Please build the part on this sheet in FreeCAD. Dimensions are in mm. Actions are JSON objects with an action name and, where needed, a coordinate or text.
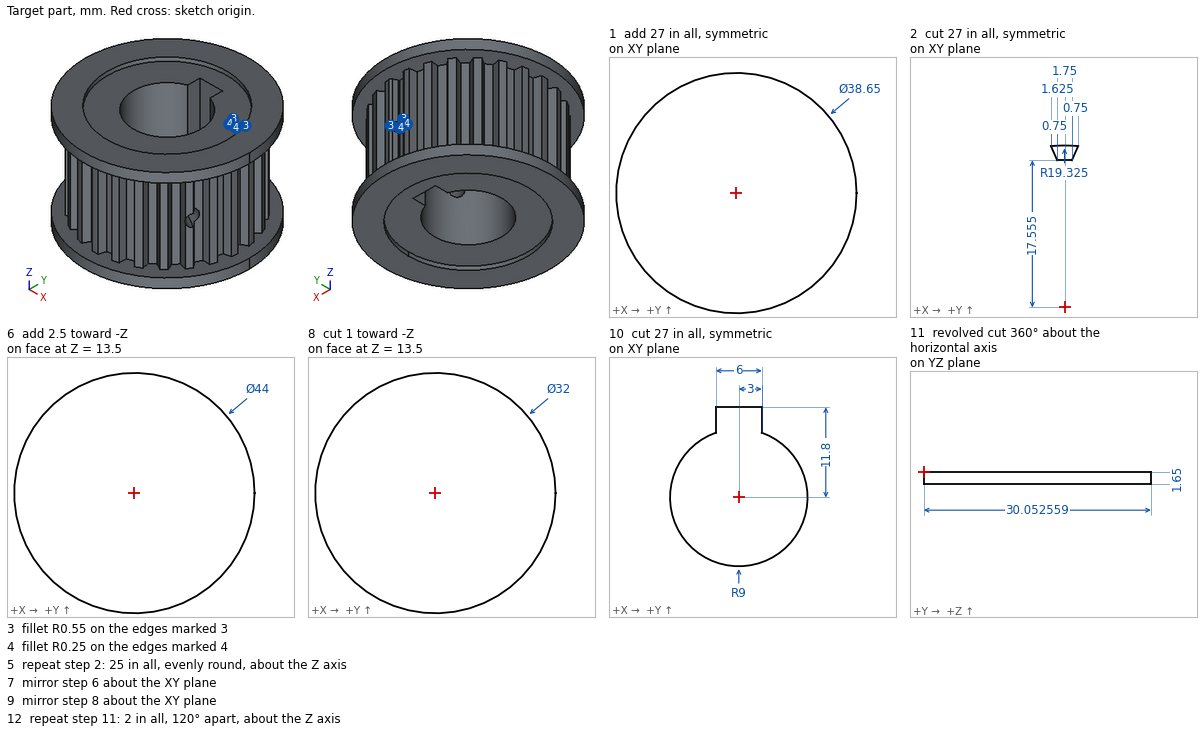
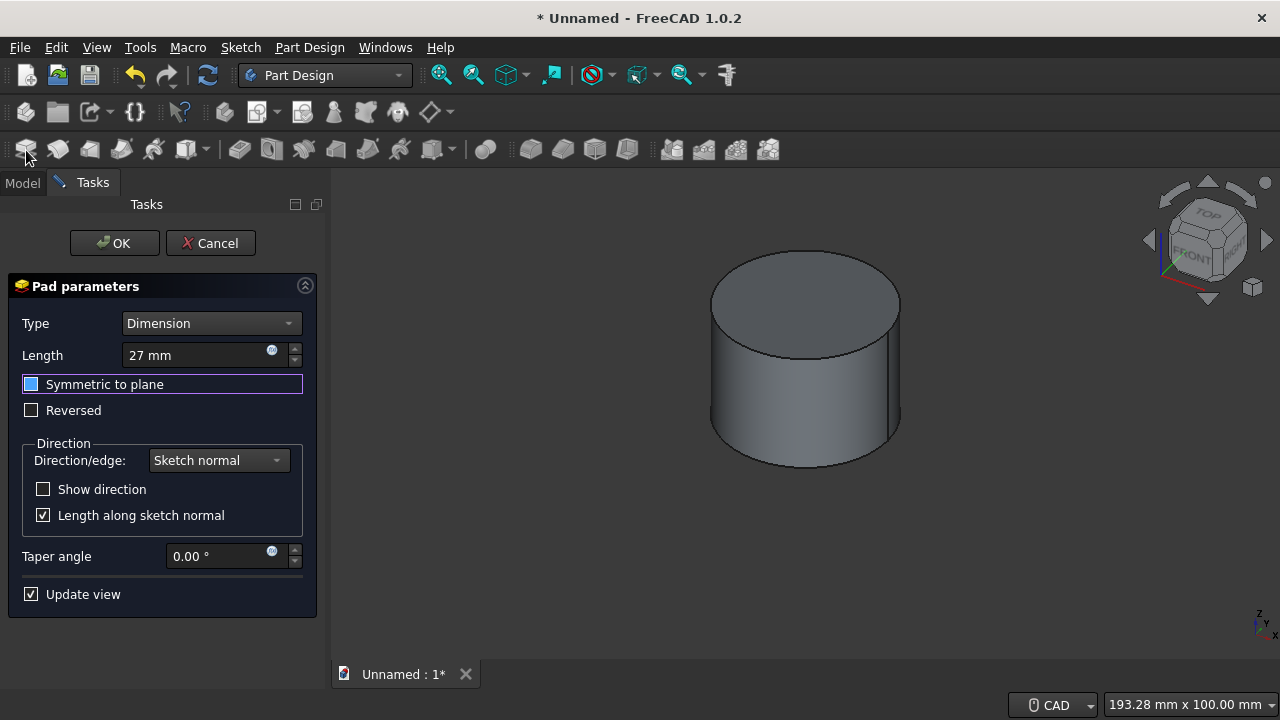
{"action": "left_click", "coordinate": [30, 384]}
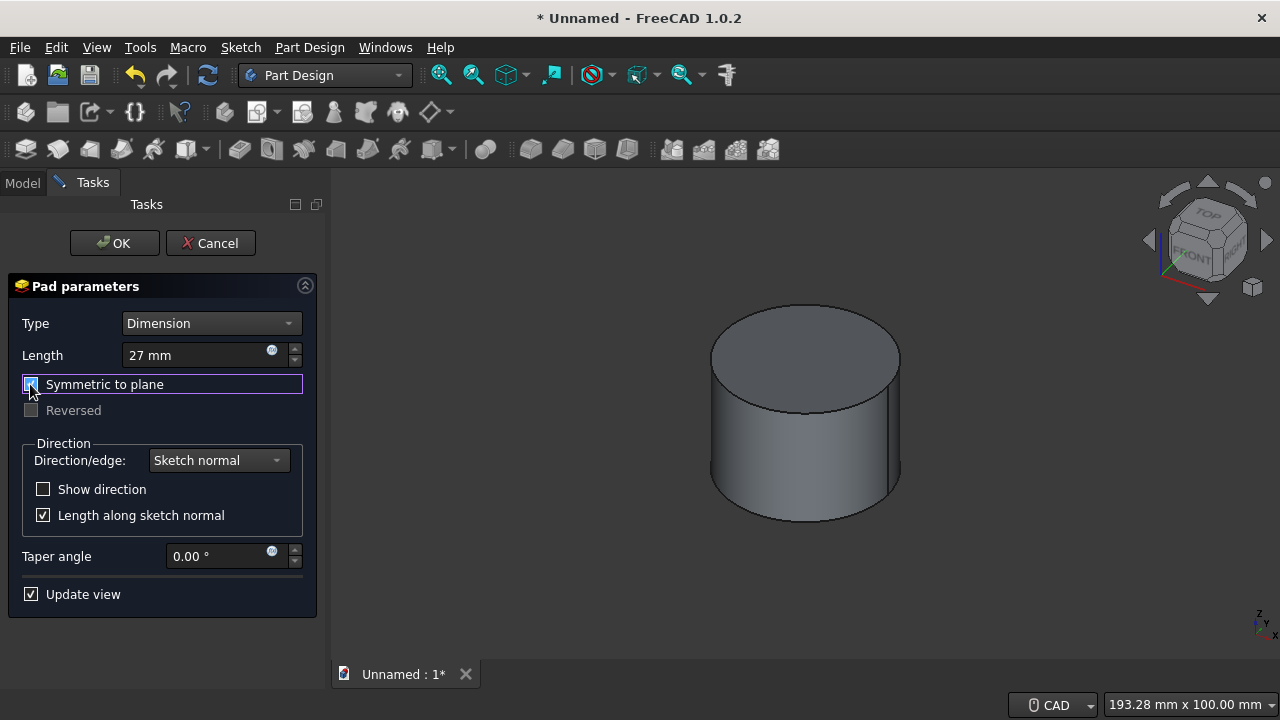
{"action": "left_click", "coordinate": [115, 243]}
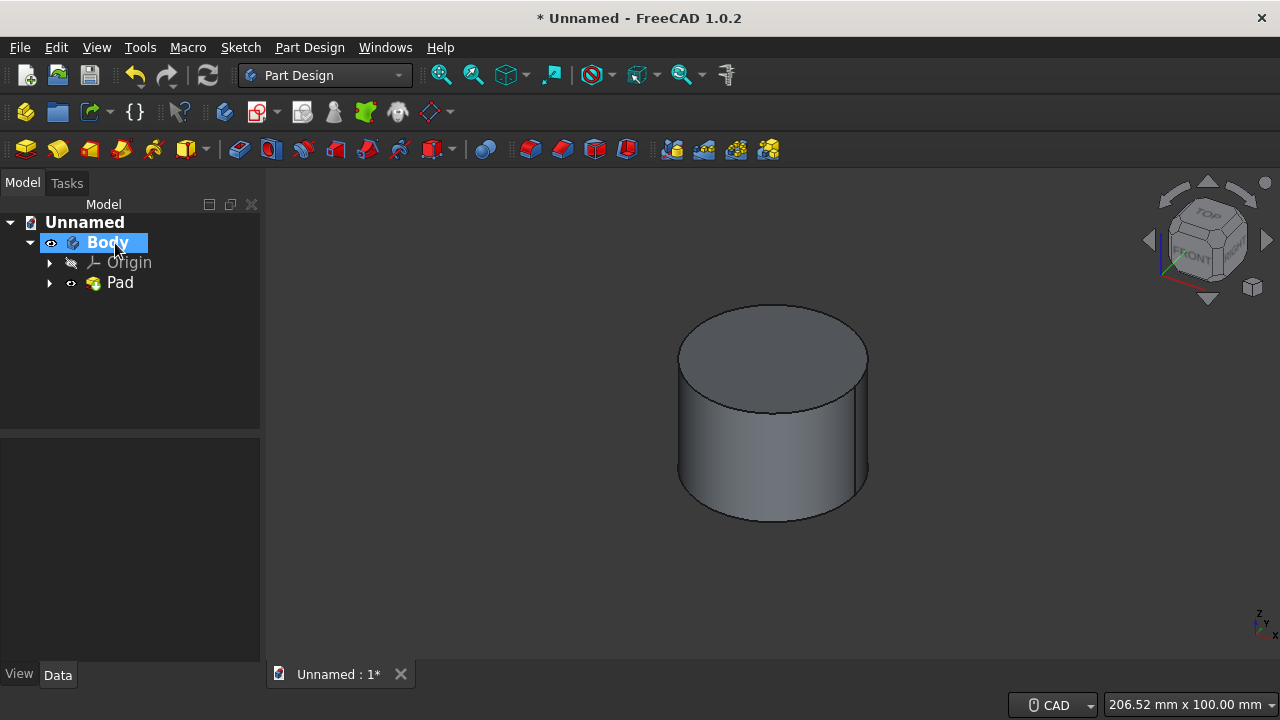
{"action": "left_click", "coordinate": [258, 112]}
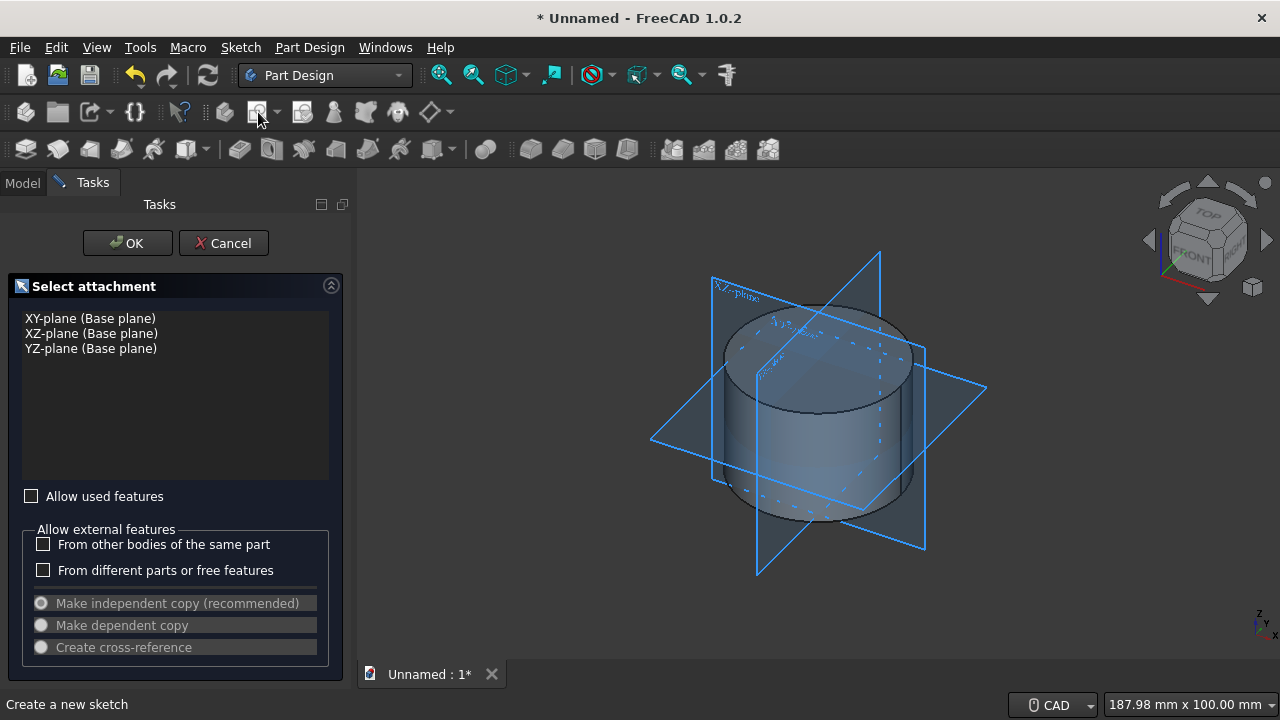
{"action": "left_click", "coordinate": [82, 318]}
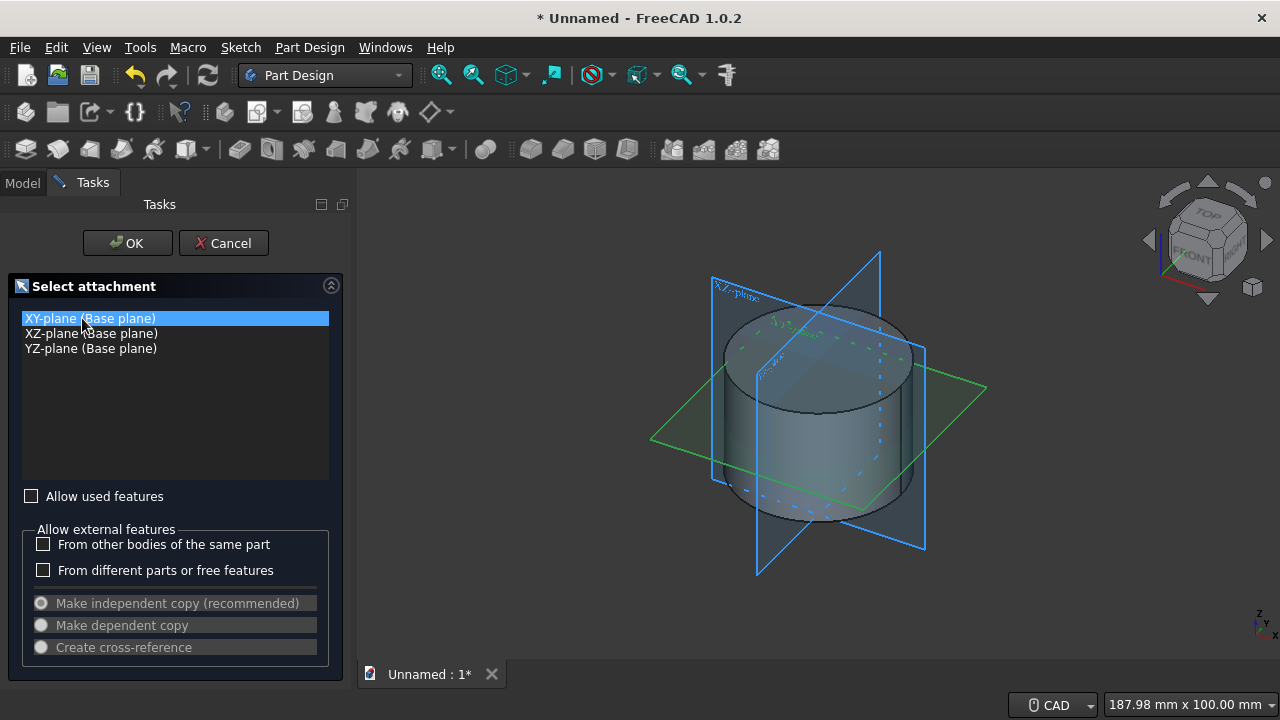
{"action": "left_click", "coordinate": [128, 243]}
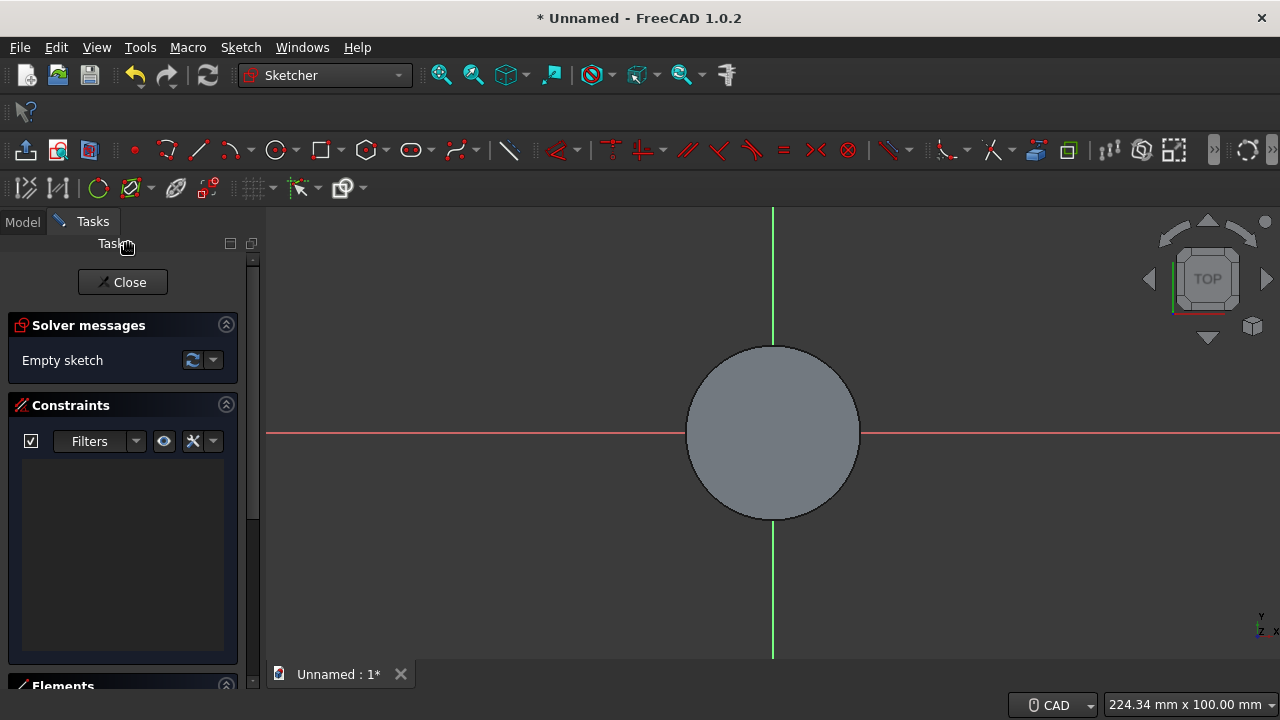
{"action": "left_click", "coordinate": [90, 150]}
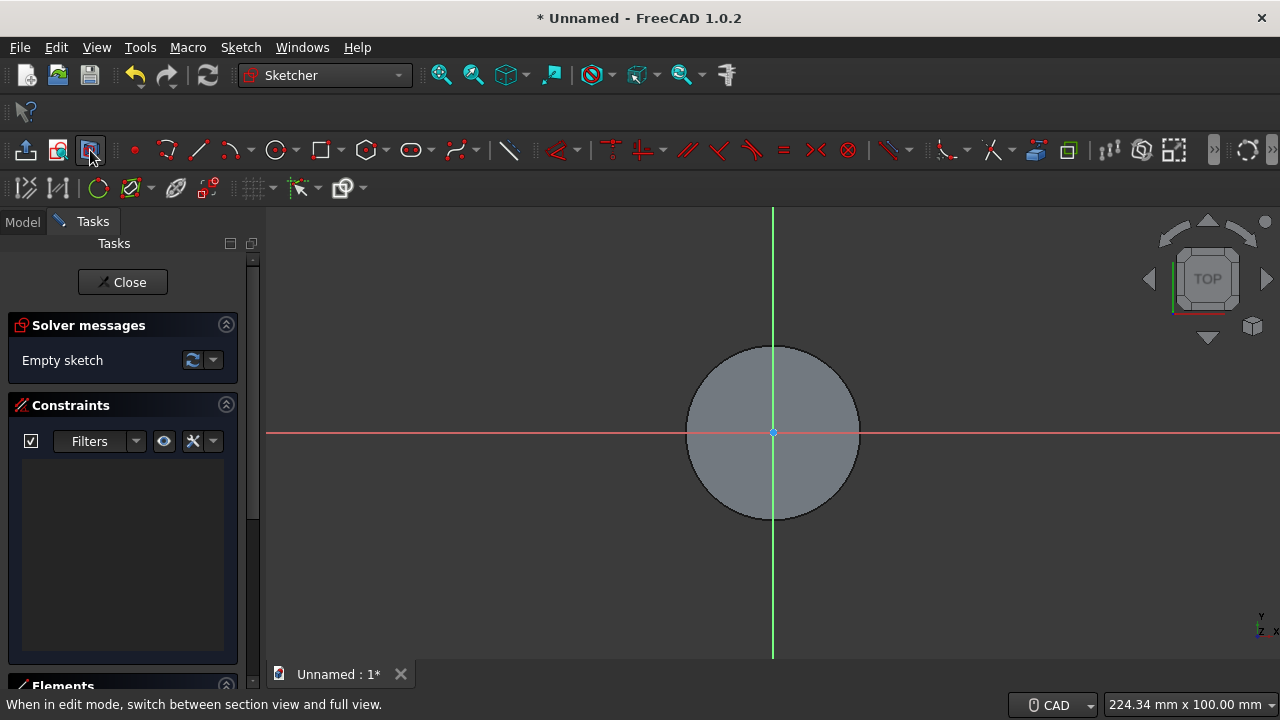
{"action": "scroll", "coordinate": [777, 345], "scroll_direction": "up", "scroll_amount": 15}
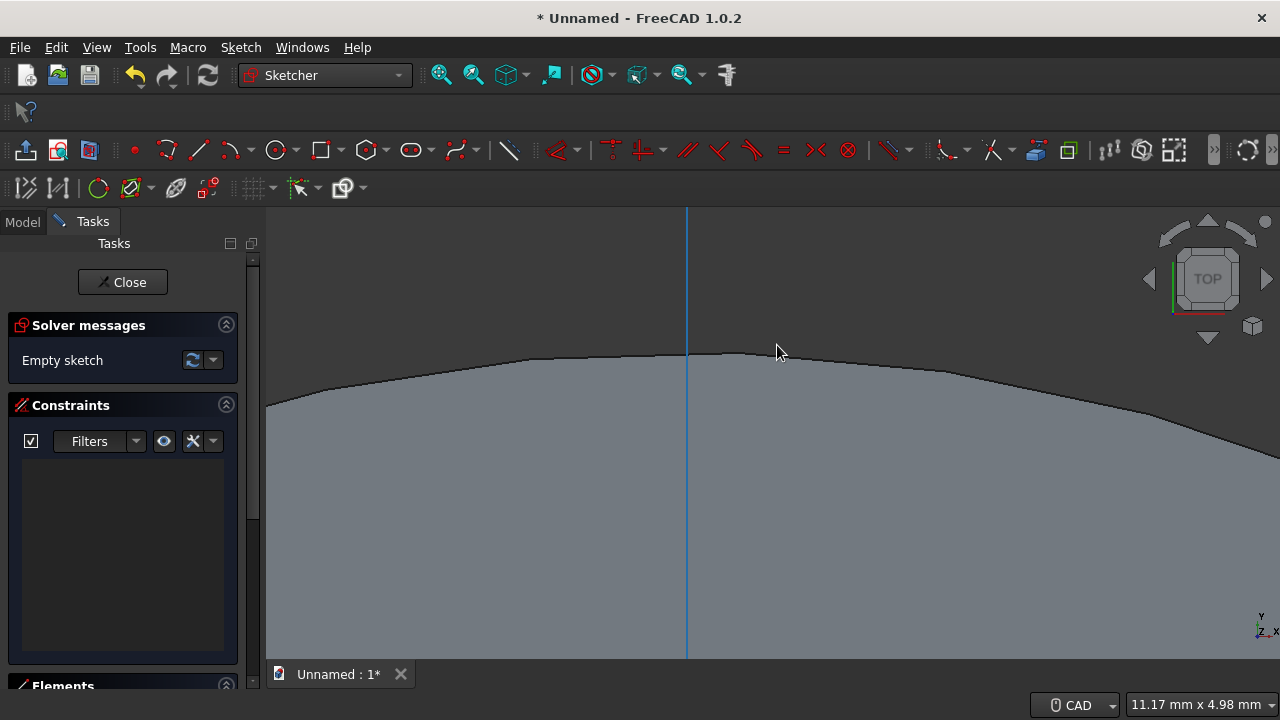
{"action": "scroll", "coordinate": [666, 432], "scroll_direction": "up", "scroll_amount": 3}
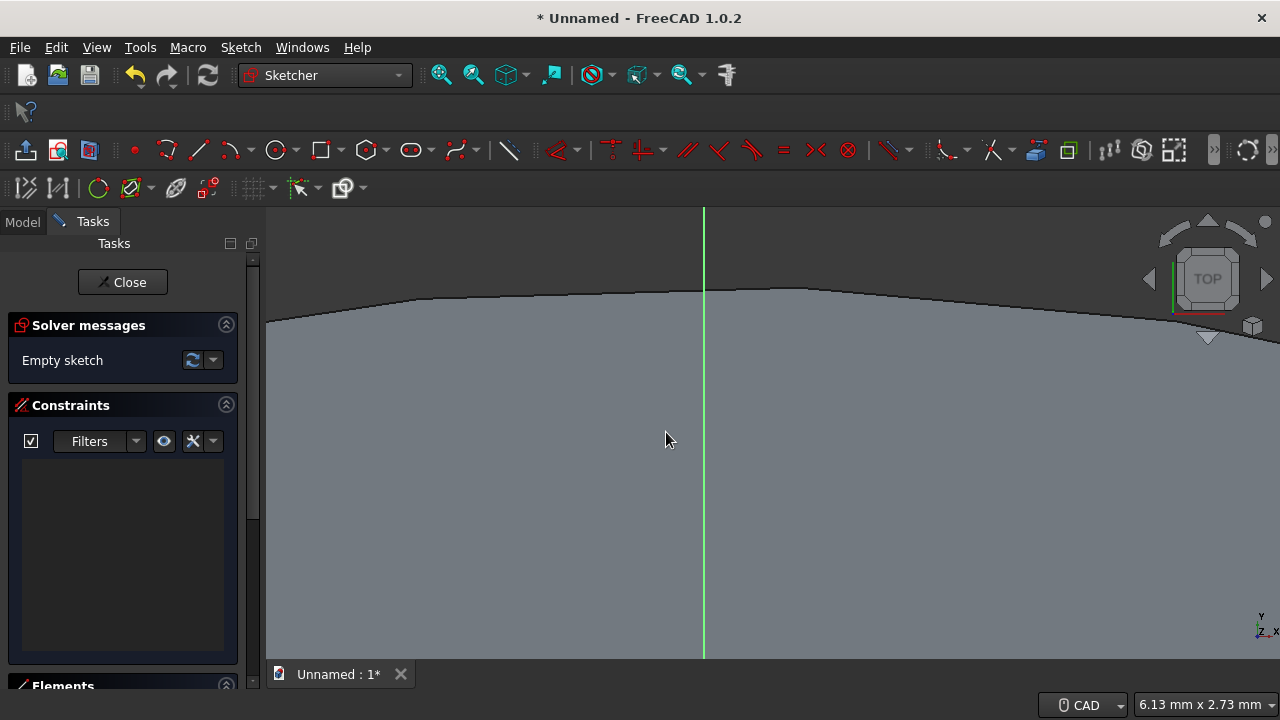
{"action": "left_click", "coordinate": [168, 150]}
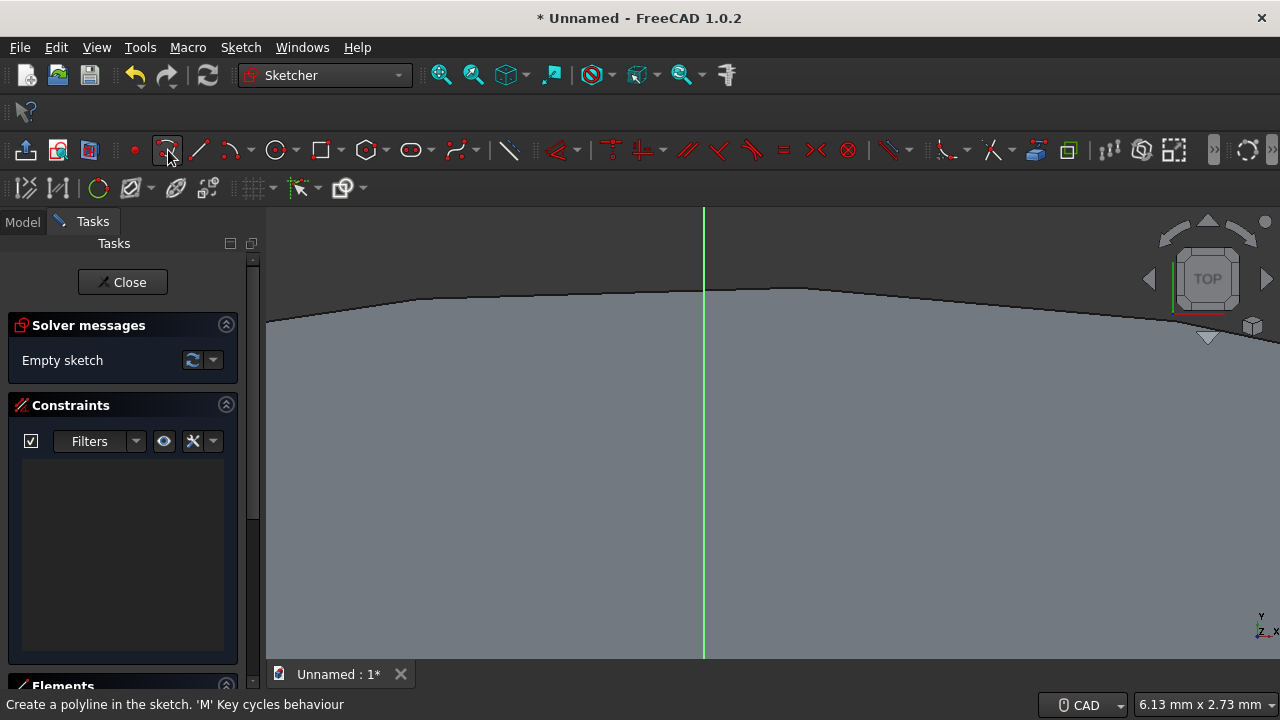
{"action": "left_click", "coordinate": [435, 298]}
{"action": "left_click", "coordinate": [559, 579]}
{"action": "left_click", "coordinate": [849, 579]}
{"action": "left_click", "coordinate": [973, 298]}
{"action": "right_click", "coordinate": [973, 298]}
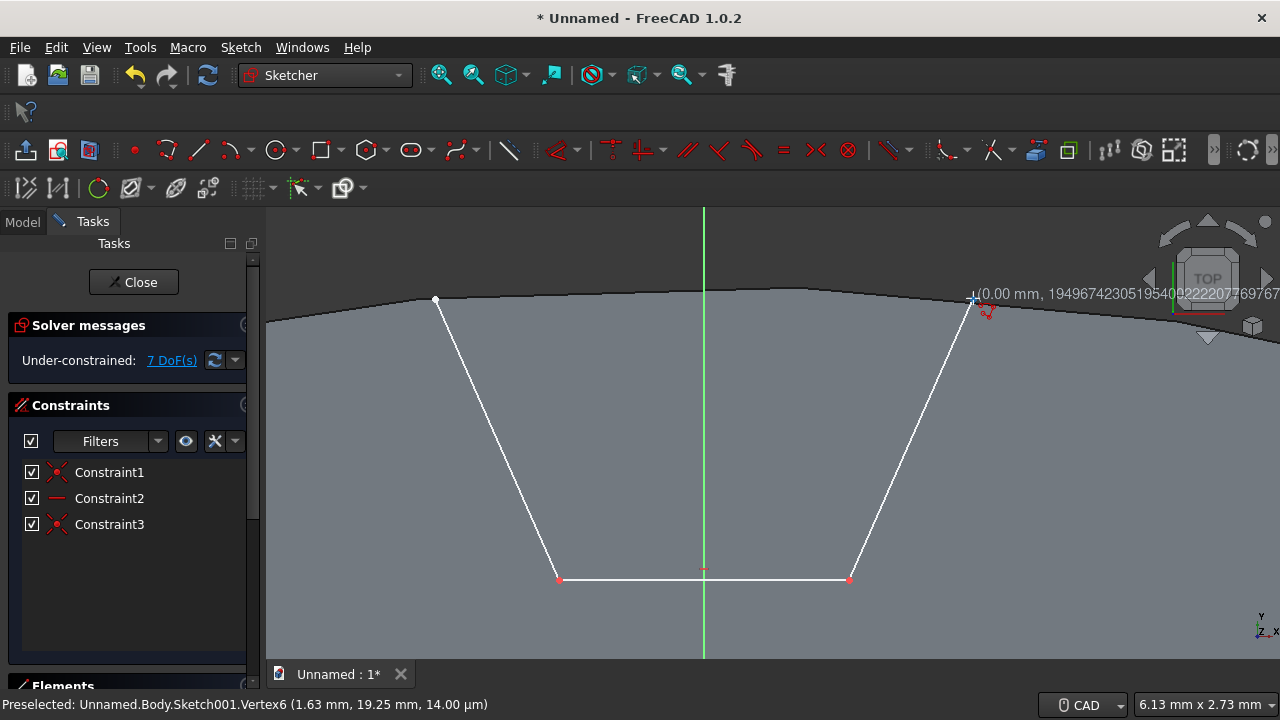
{"action": "key", "text": "g 3 a"}